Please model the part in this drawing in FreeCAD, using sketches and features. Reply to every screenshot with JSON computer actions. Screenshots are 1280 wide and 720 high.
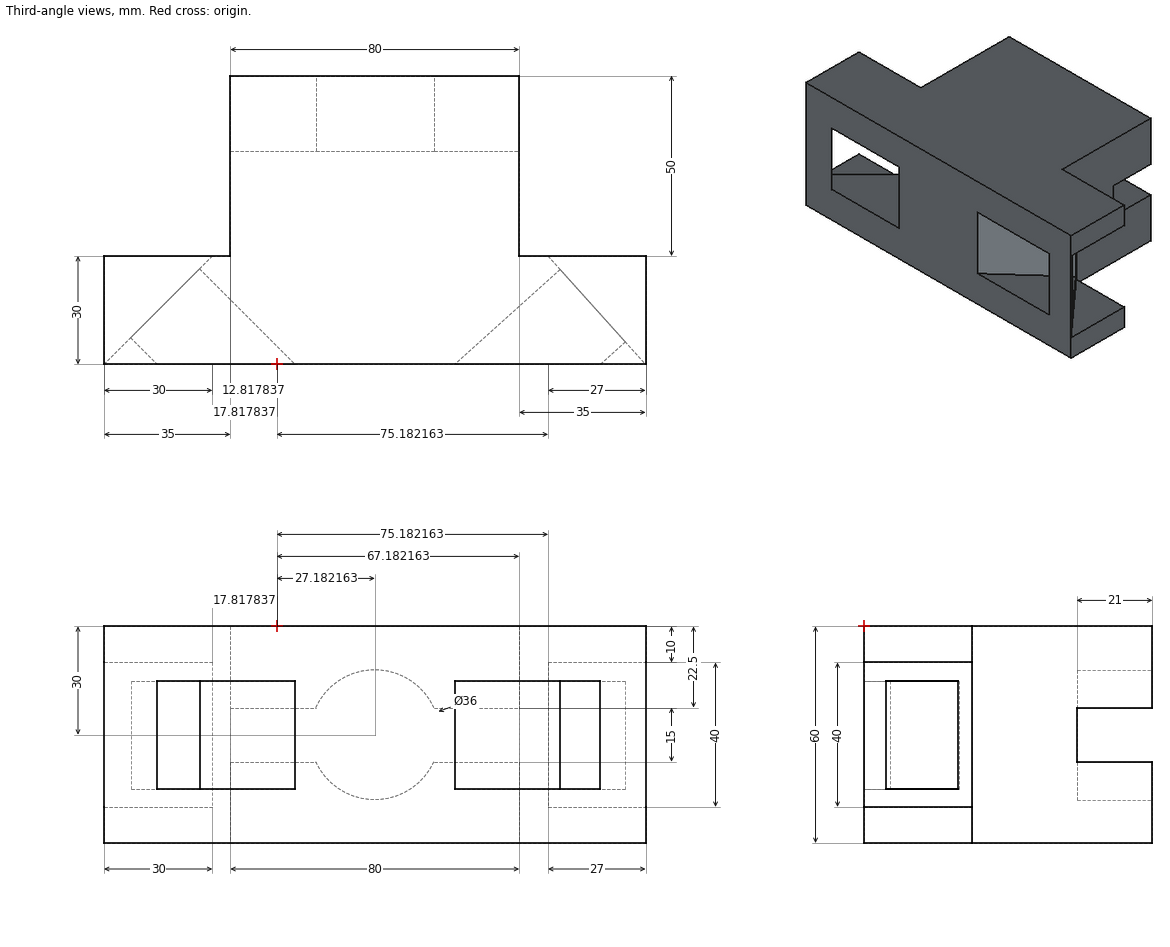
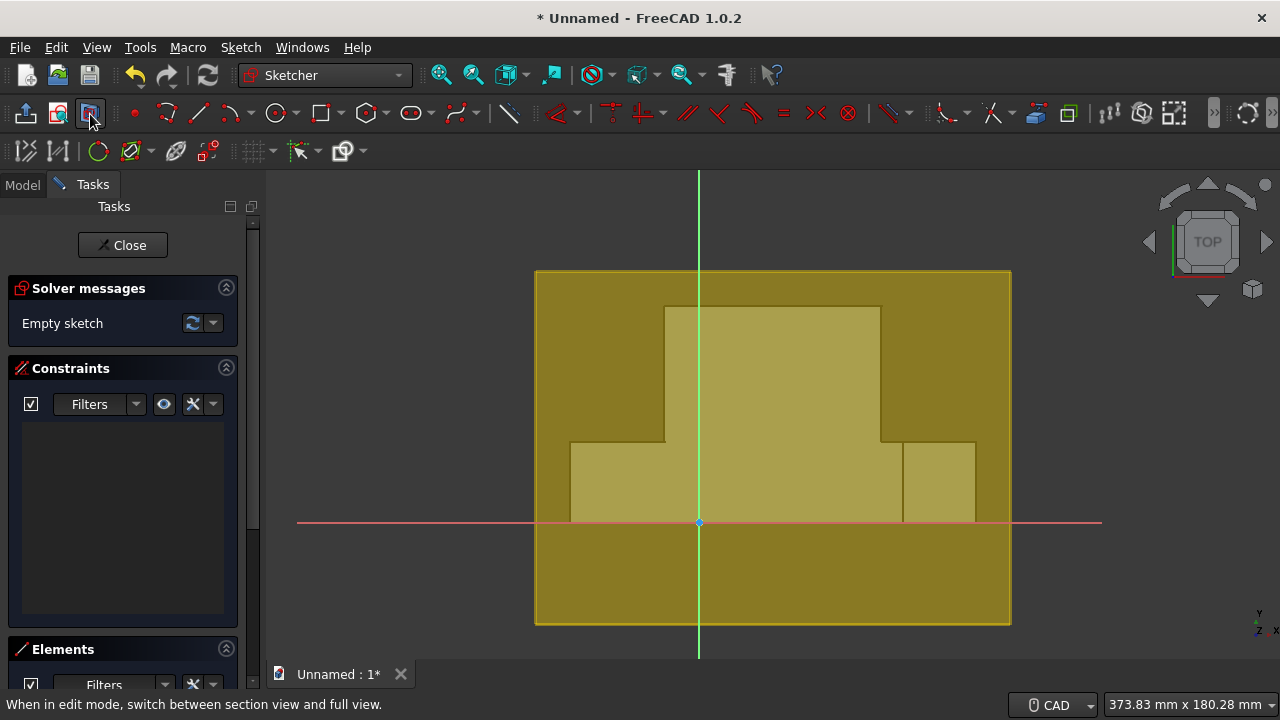
{"action": "scroll", "coordinate": [1017, 505], "scroll_direction": "up", "scroll_amount": 7}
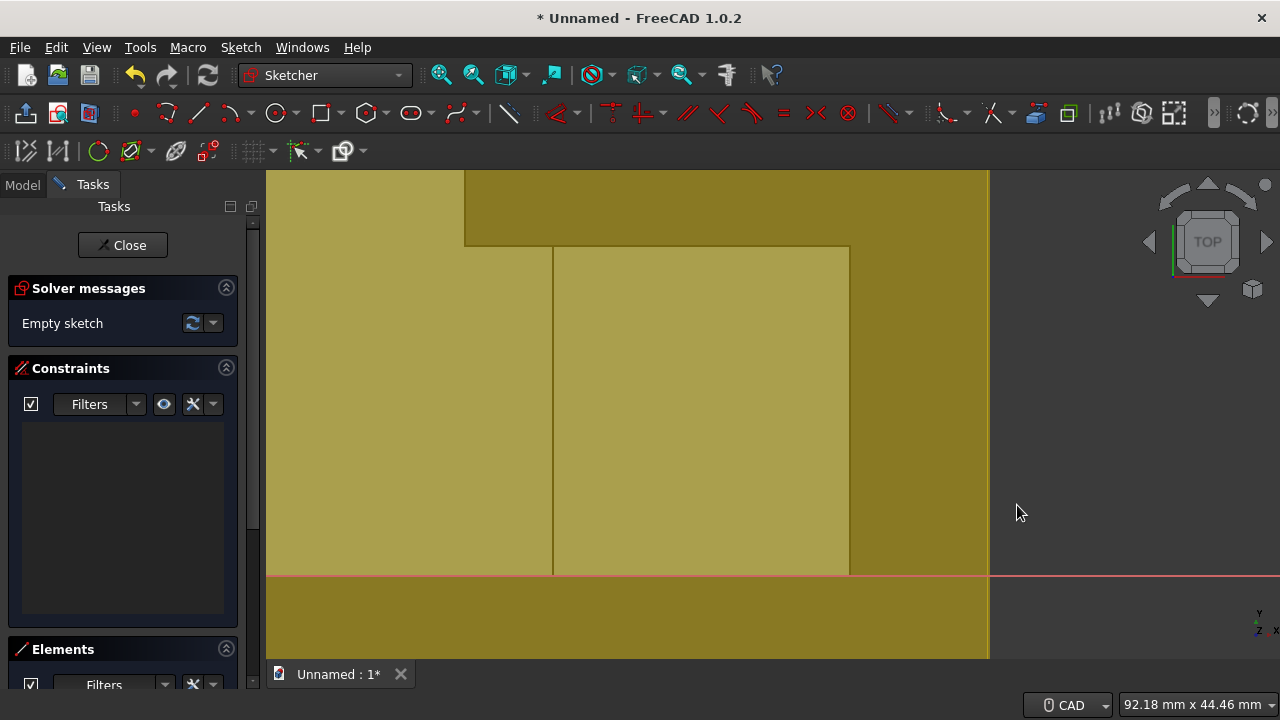
{"action": "left_click", "coordinate": [168, 114]}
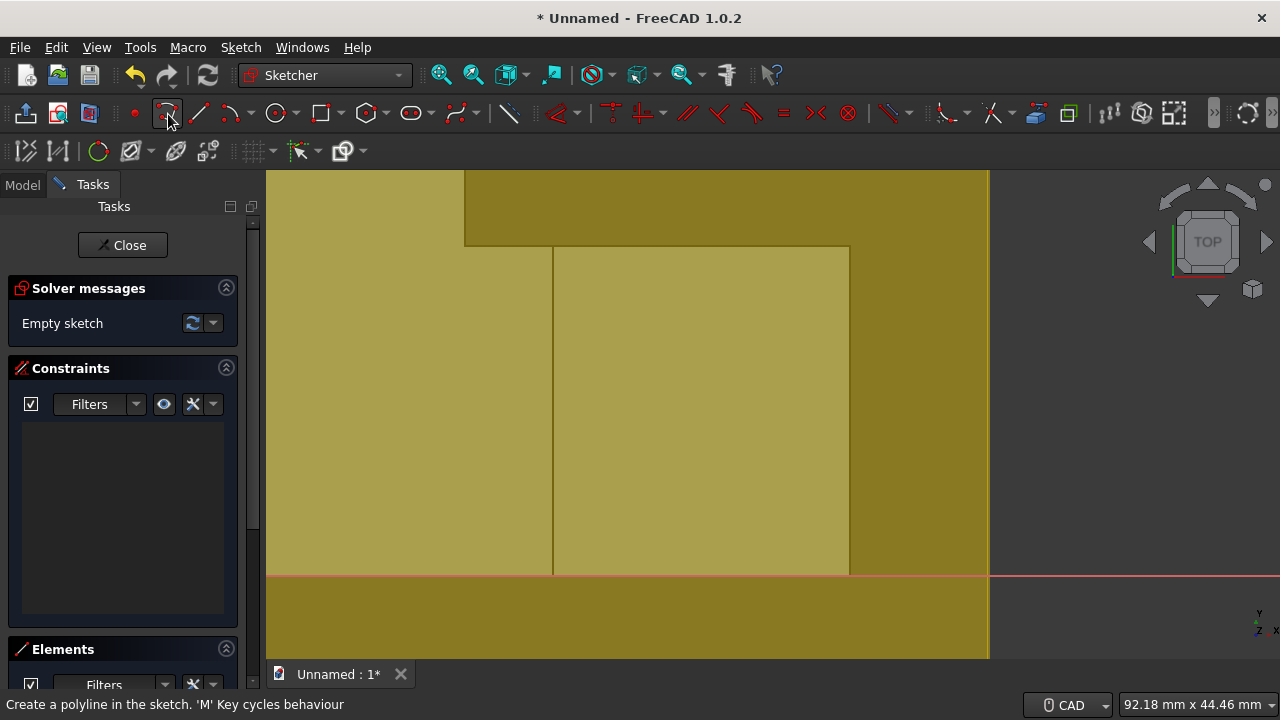
{"action": "left_click", "coordinate": [553, 576]}
{"action": "left_click", "coordinate": [850, 567]}
{"action": "left_click", "coordinate": [553, 246]}
{"action": "left_click", "coordinate": [553, 576]}
{"action": "key", "text": "Escape"}
{"action": "key", "text": "Escape"}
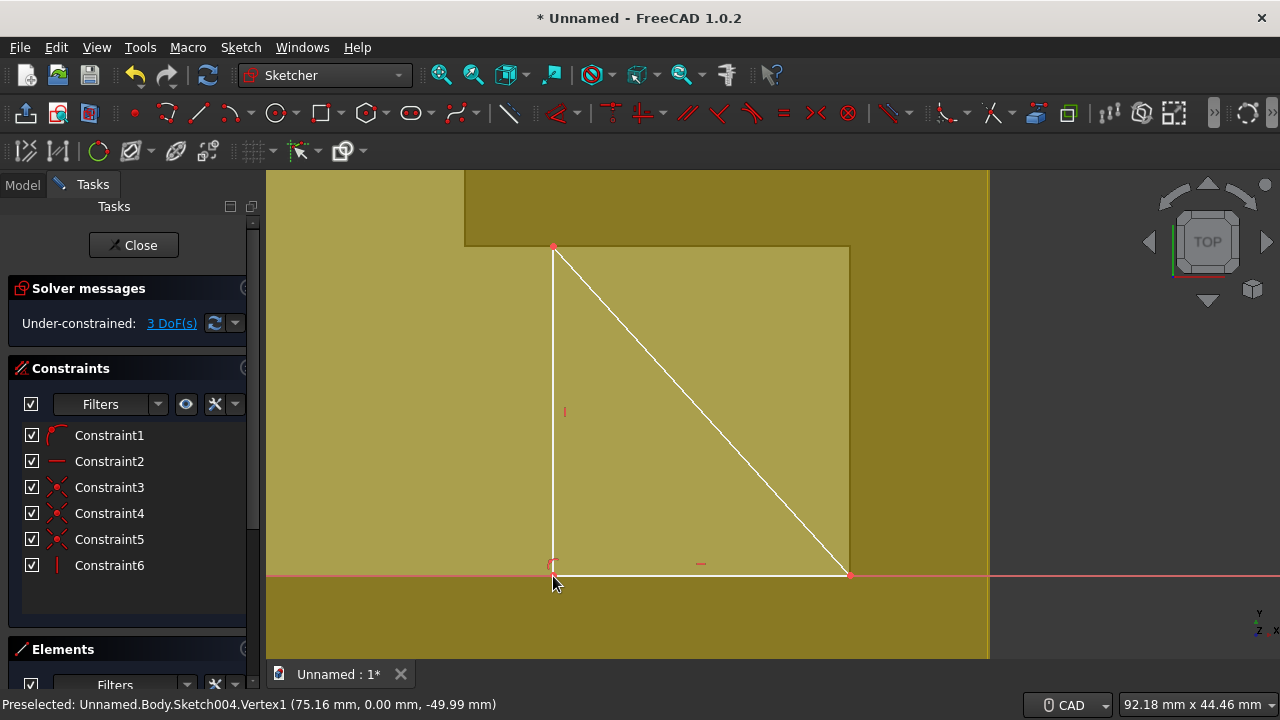
{"action": "left_click", "coordinate": [556, 114]}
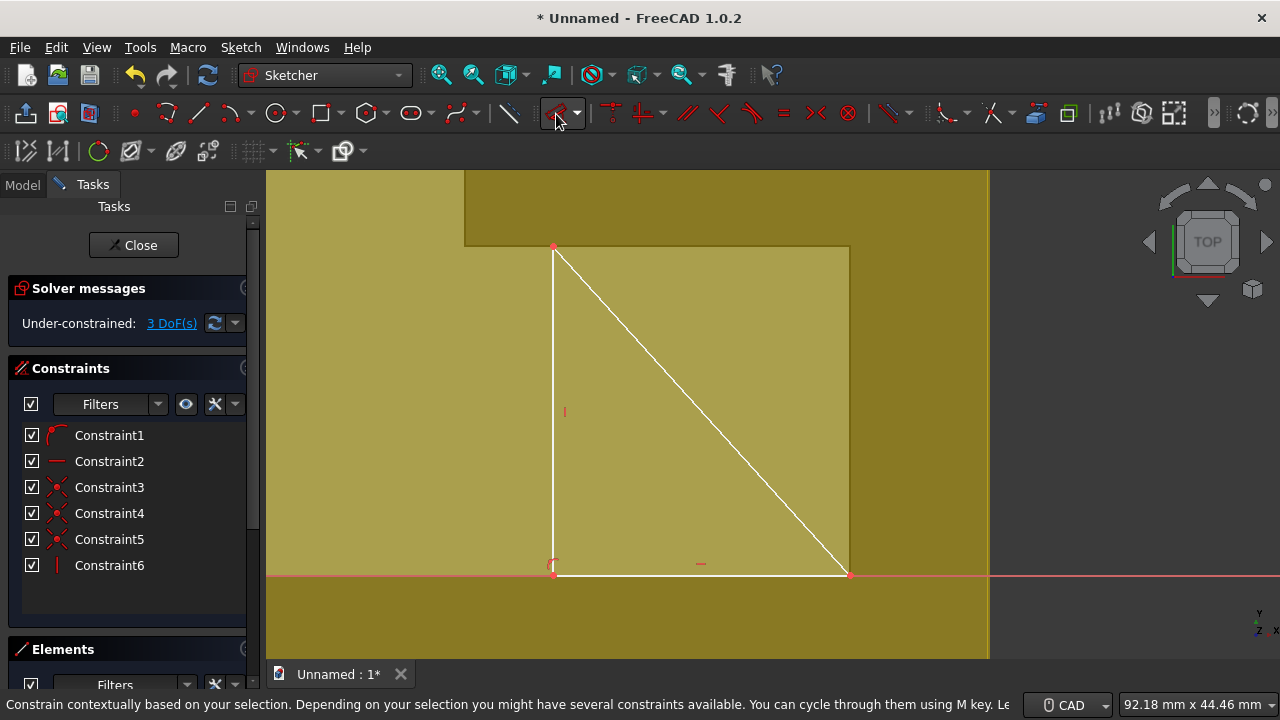
{"action": "left_click", "coordinate": [642, 576]}
{"action": "left_click", "coordinate": [702, 610]}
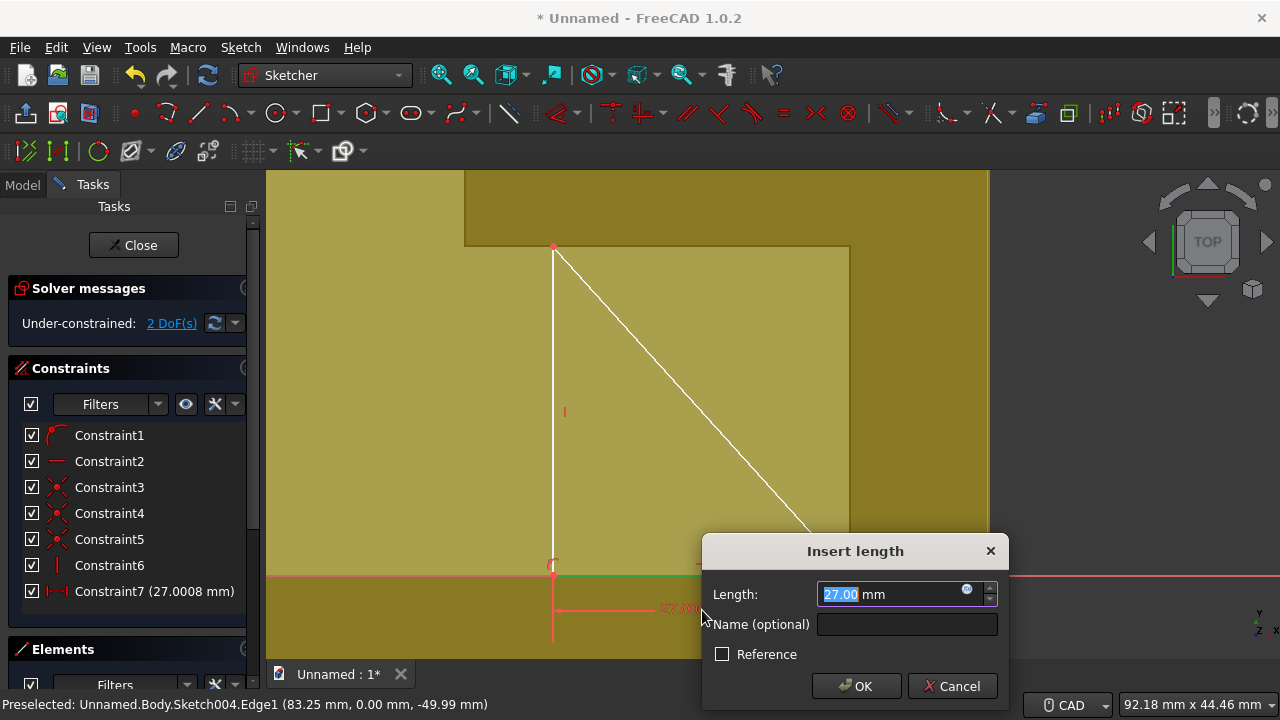
{"action": "type", "text": "27"}
{"action": "key", "text": "Return"}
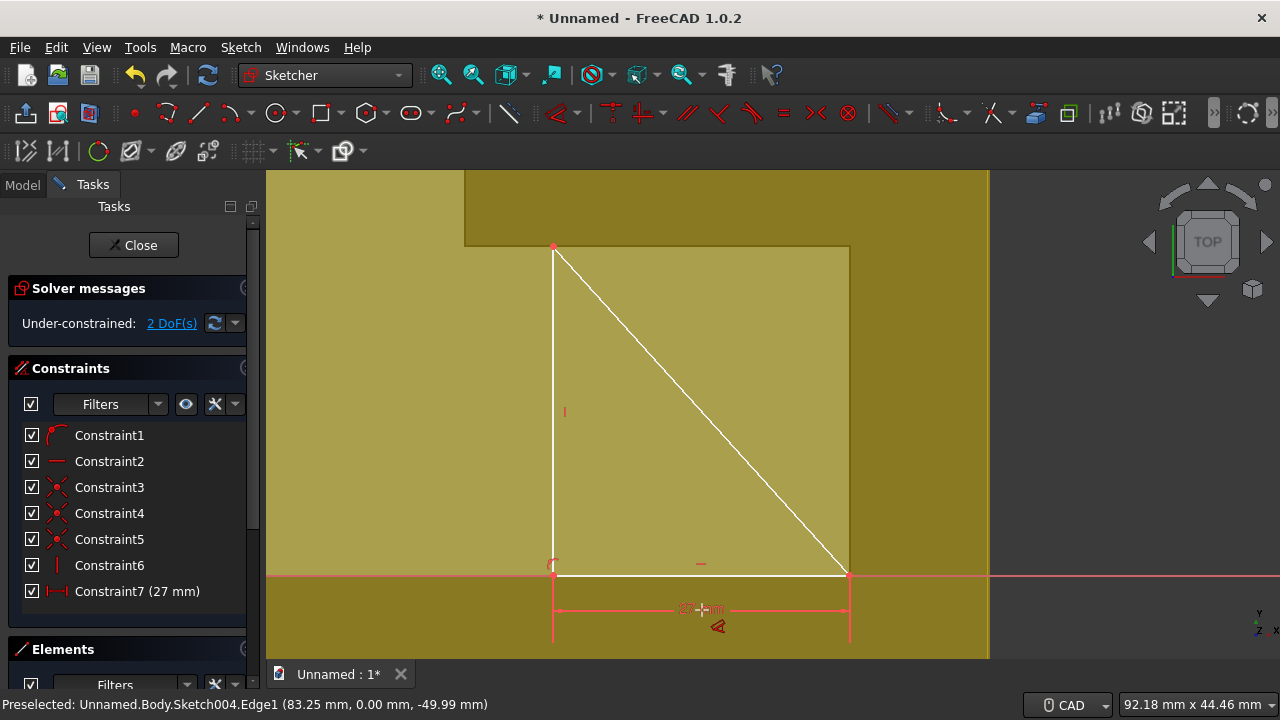
{"action": "left_click", "coordinate": [553, 346]}
{"action": "left_click", "coordinate": [519, 411]}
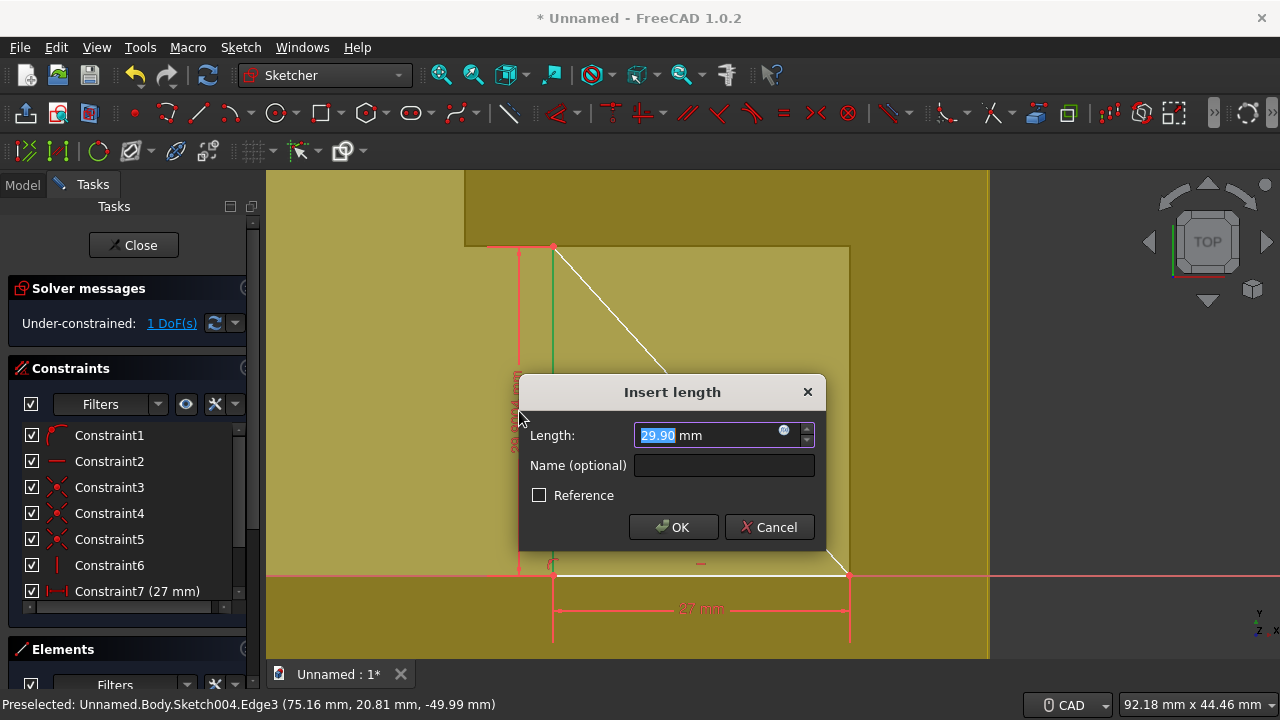
{"action": "type", "text": "30"}
{"action": "key", "text": "Return"}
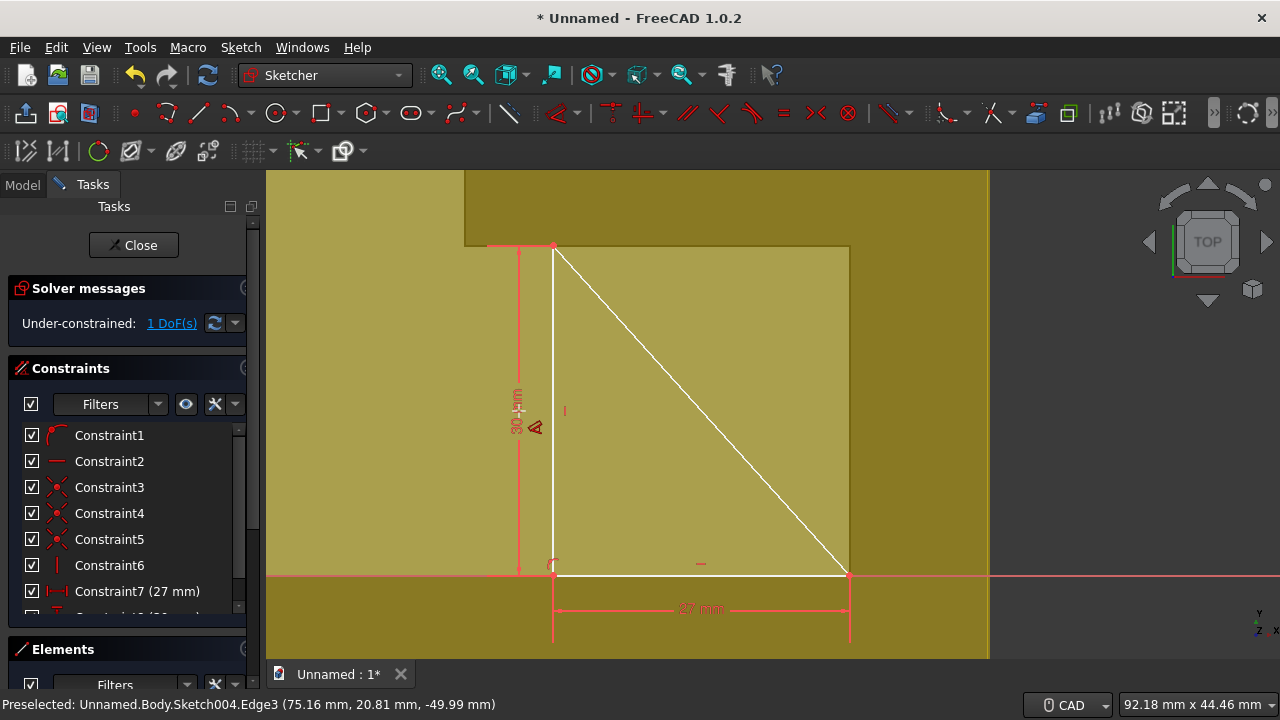
{"action": "left_click", "coordinate": [553, 576]}
{"action": "left_click", "coordinate": [424, 610]}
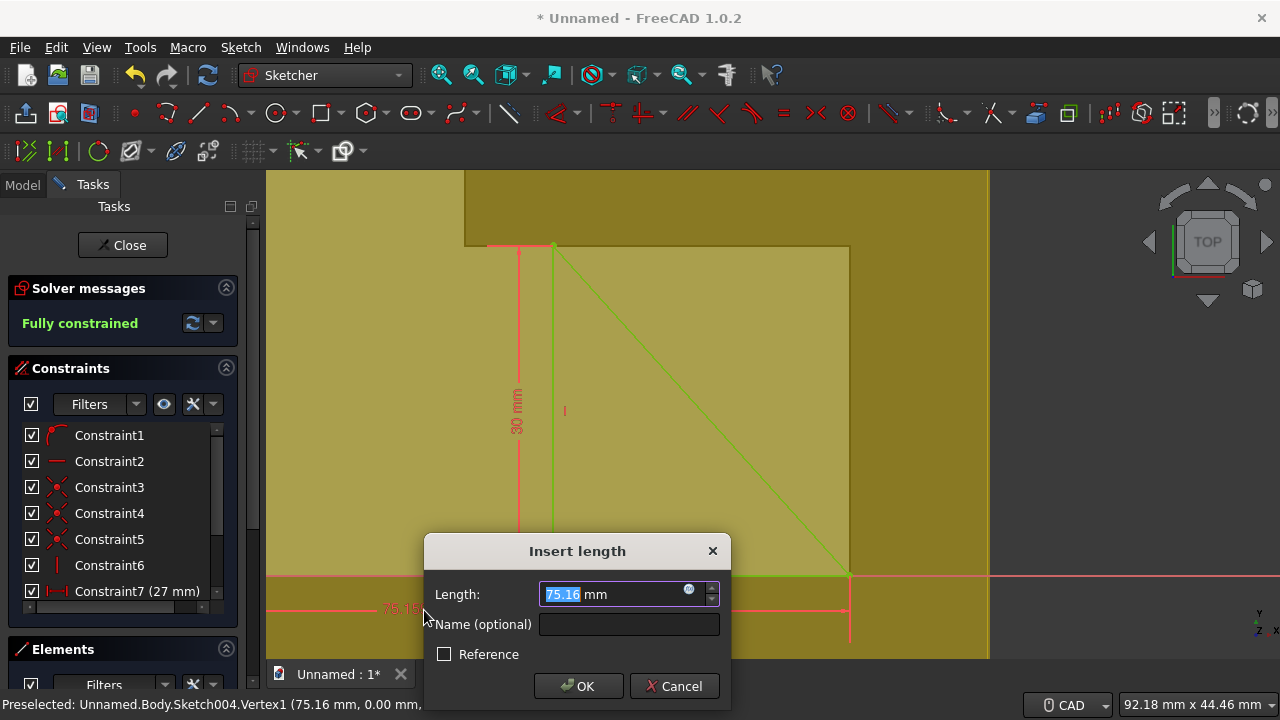
{"action": "type", "text": "75.182163"}
{"action": "key", "text": "Return"}
{"action": "key", "text": "Escape"}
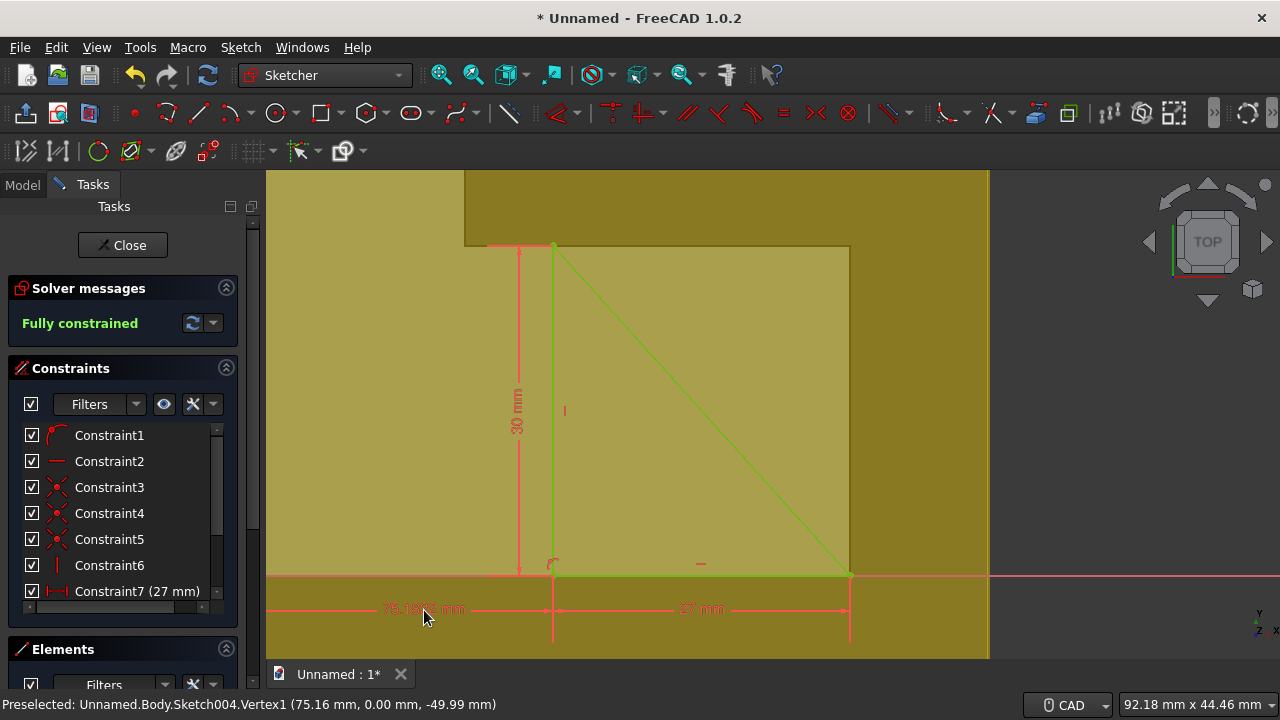
{"action": "left_click", "coordinate": [123, 245]}